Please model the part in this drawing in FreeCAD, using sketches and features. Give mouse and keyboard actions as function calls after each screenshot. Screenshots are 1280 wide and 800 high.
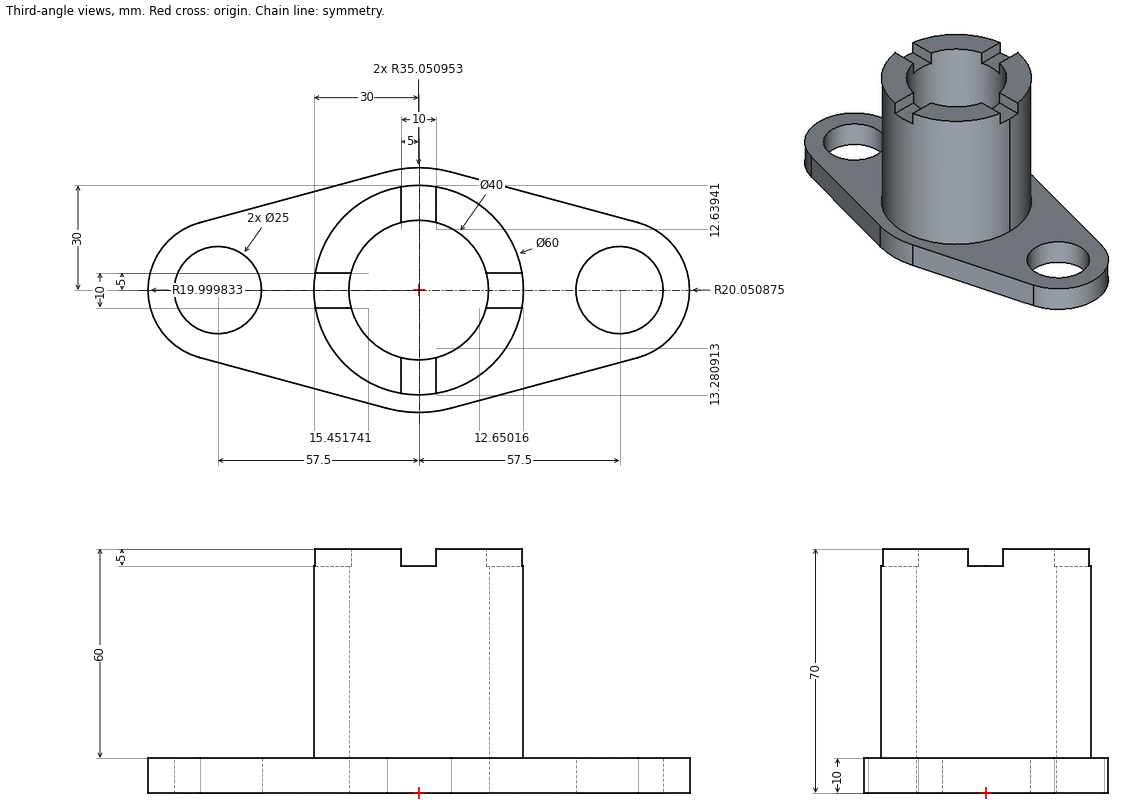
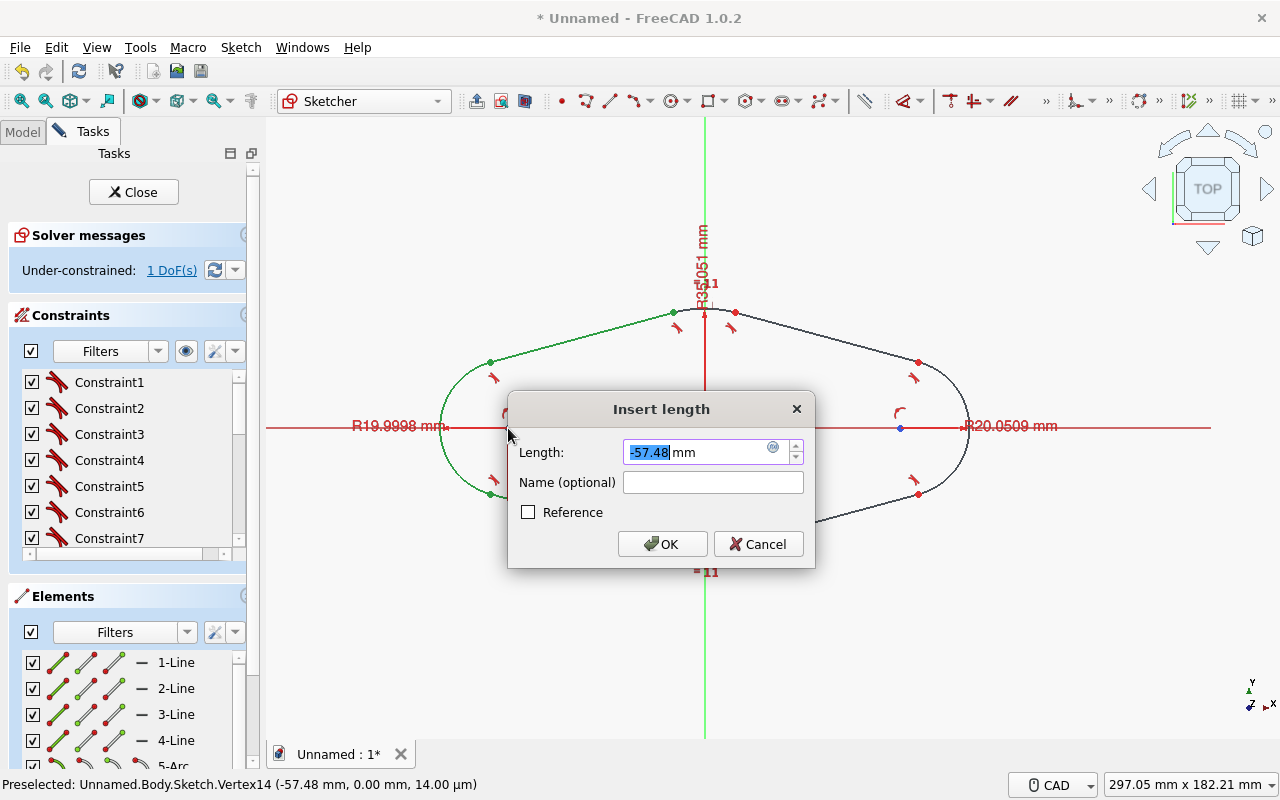
text(-57.5)
key(Return)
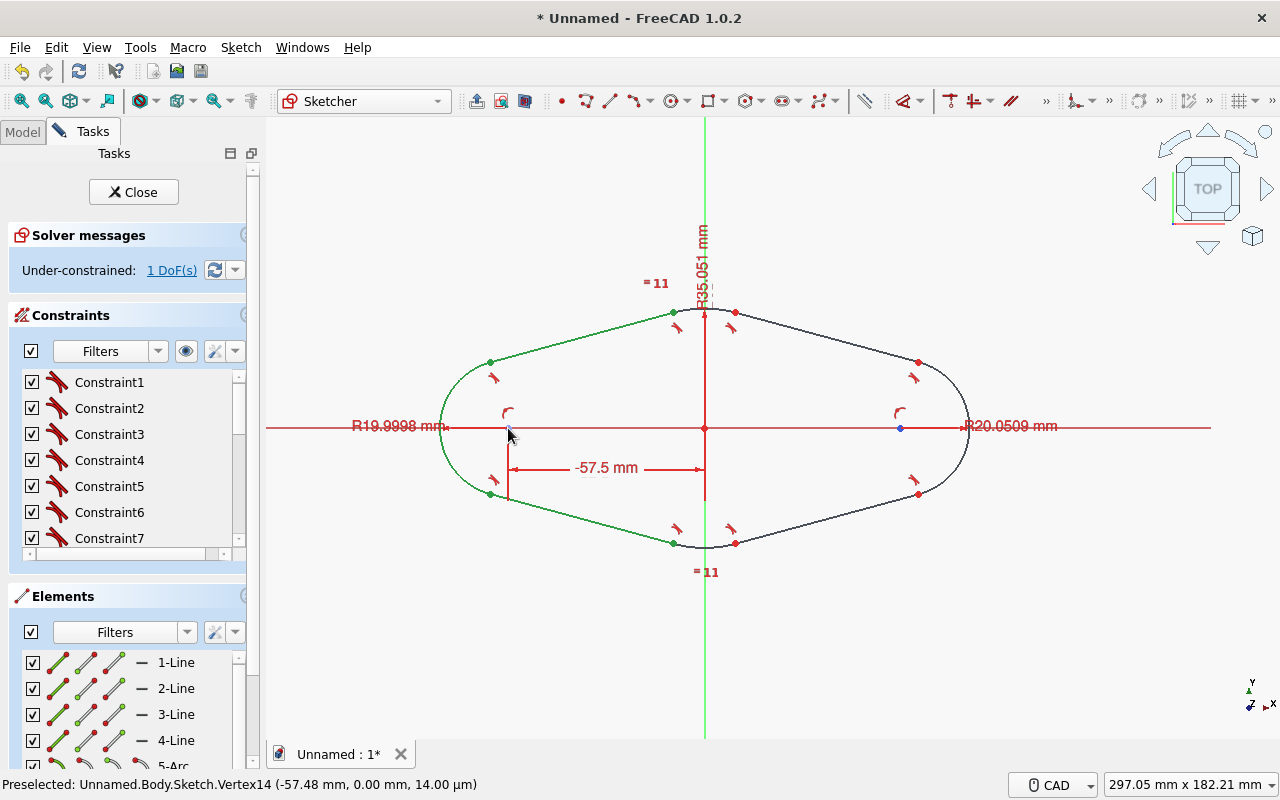
click(901, 428)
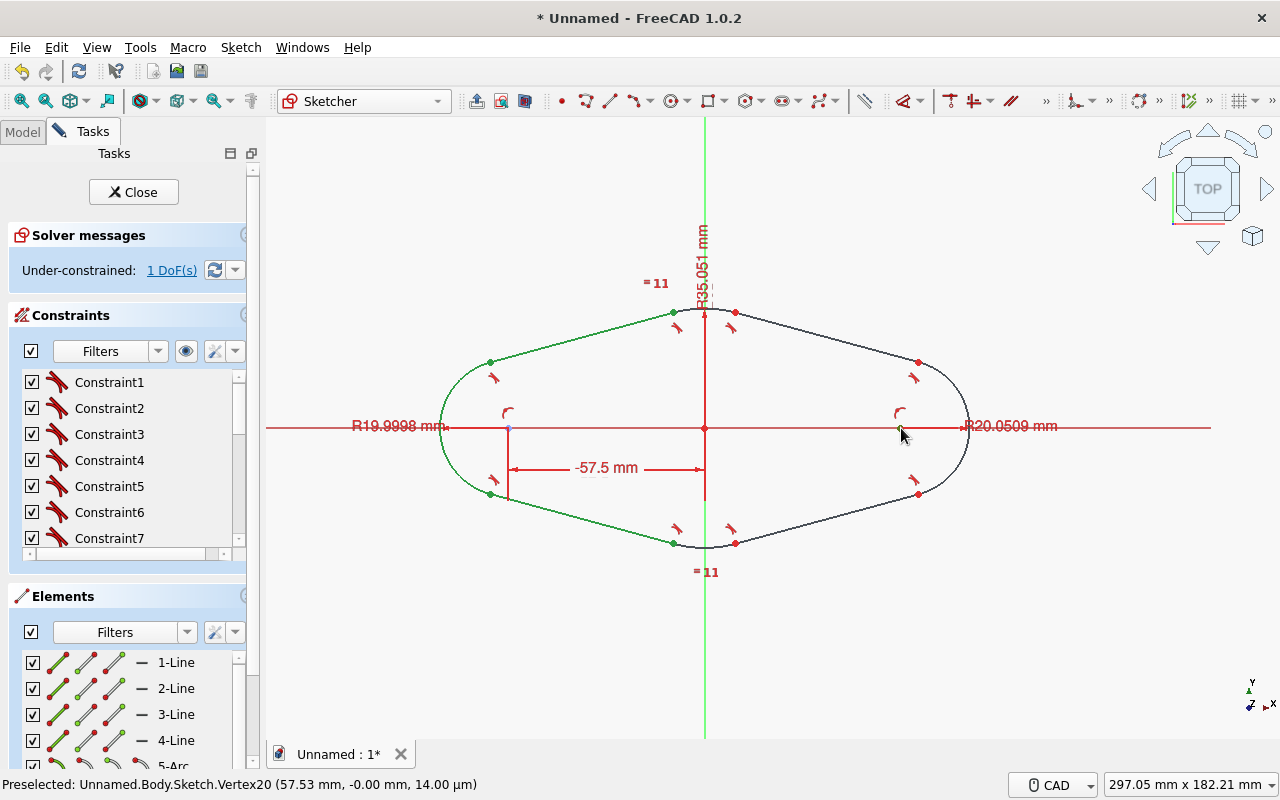
key(l)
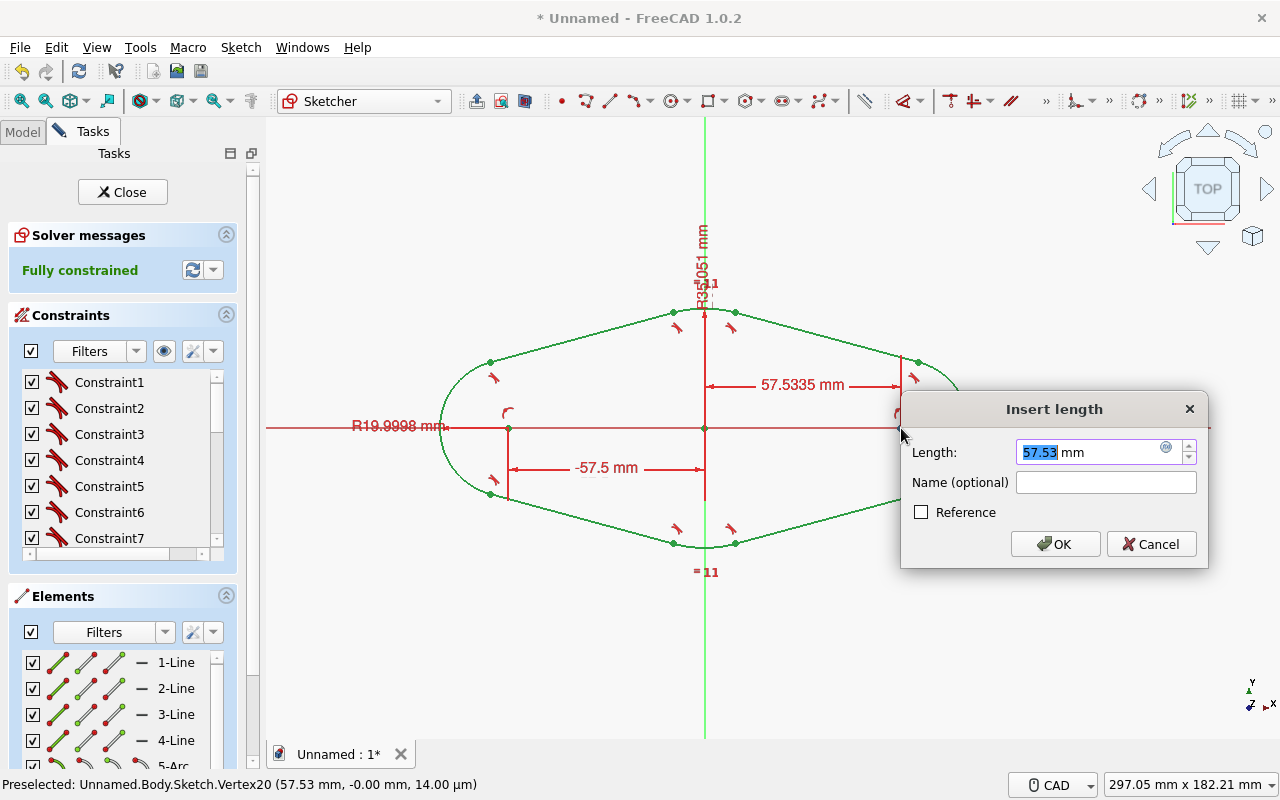
text(57.5)
key(Return)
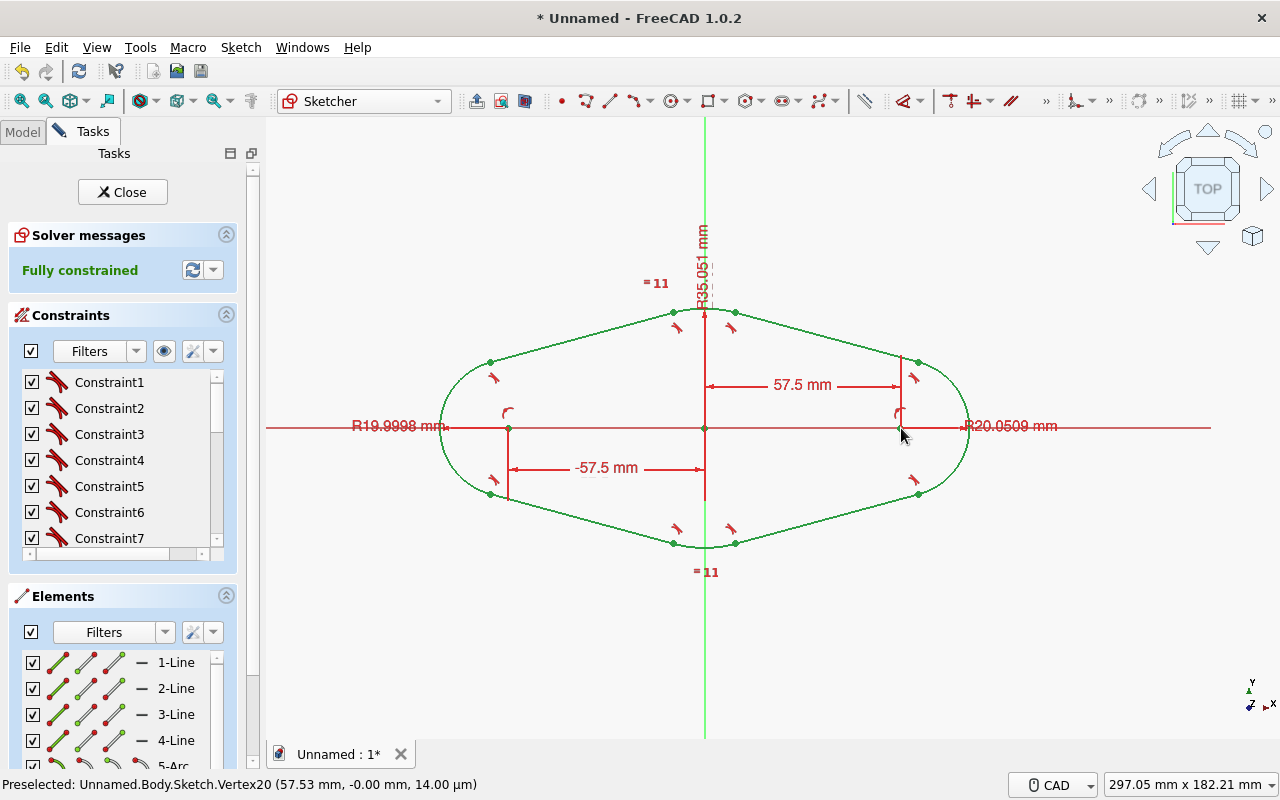
click(123, 192)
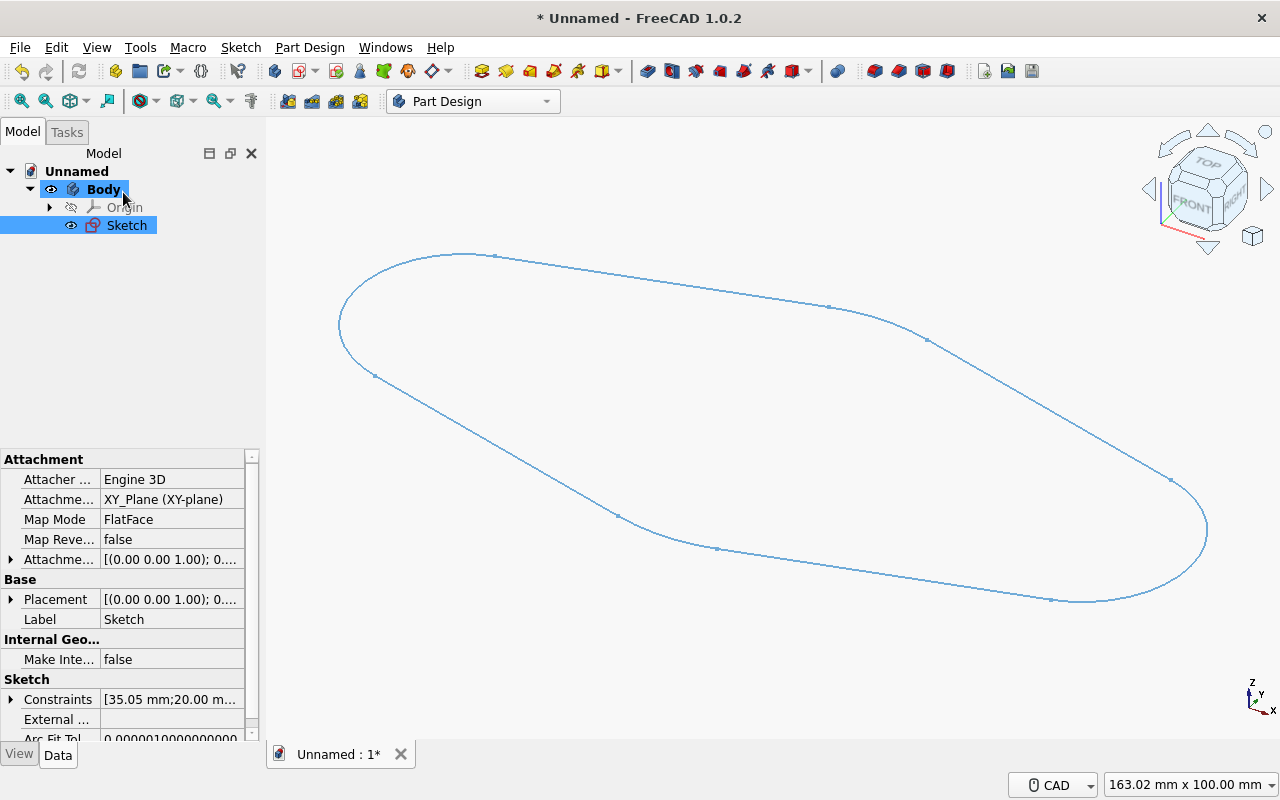
click(482, 72)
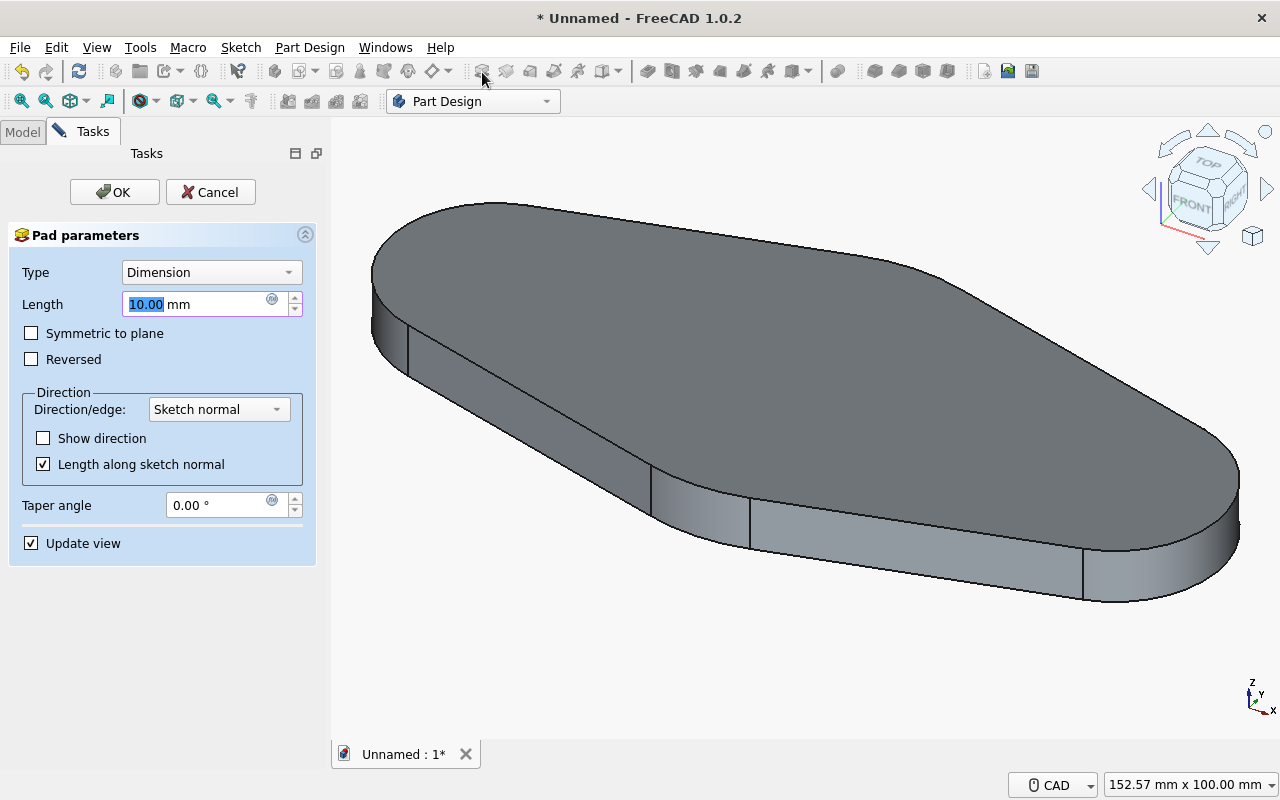
text(10)
key(Tab)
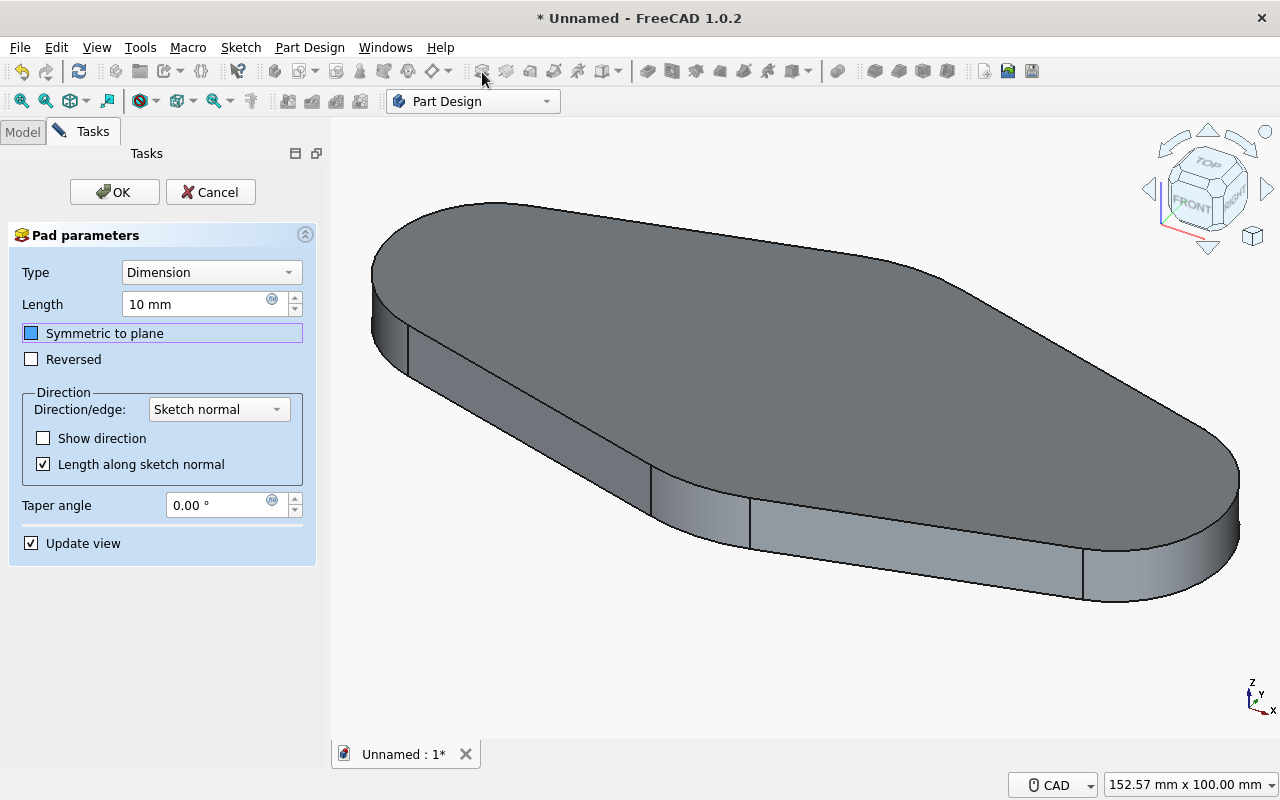
click(115, 192)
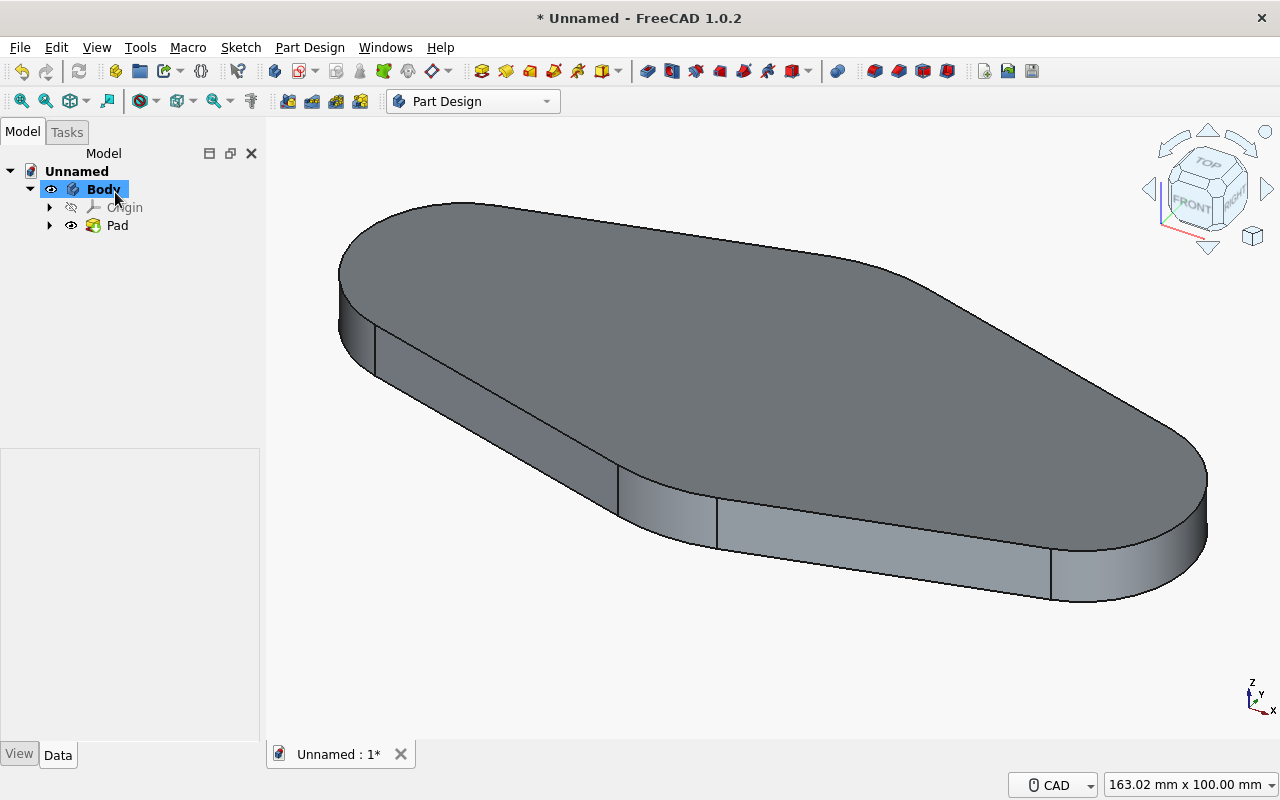
click(22, 102)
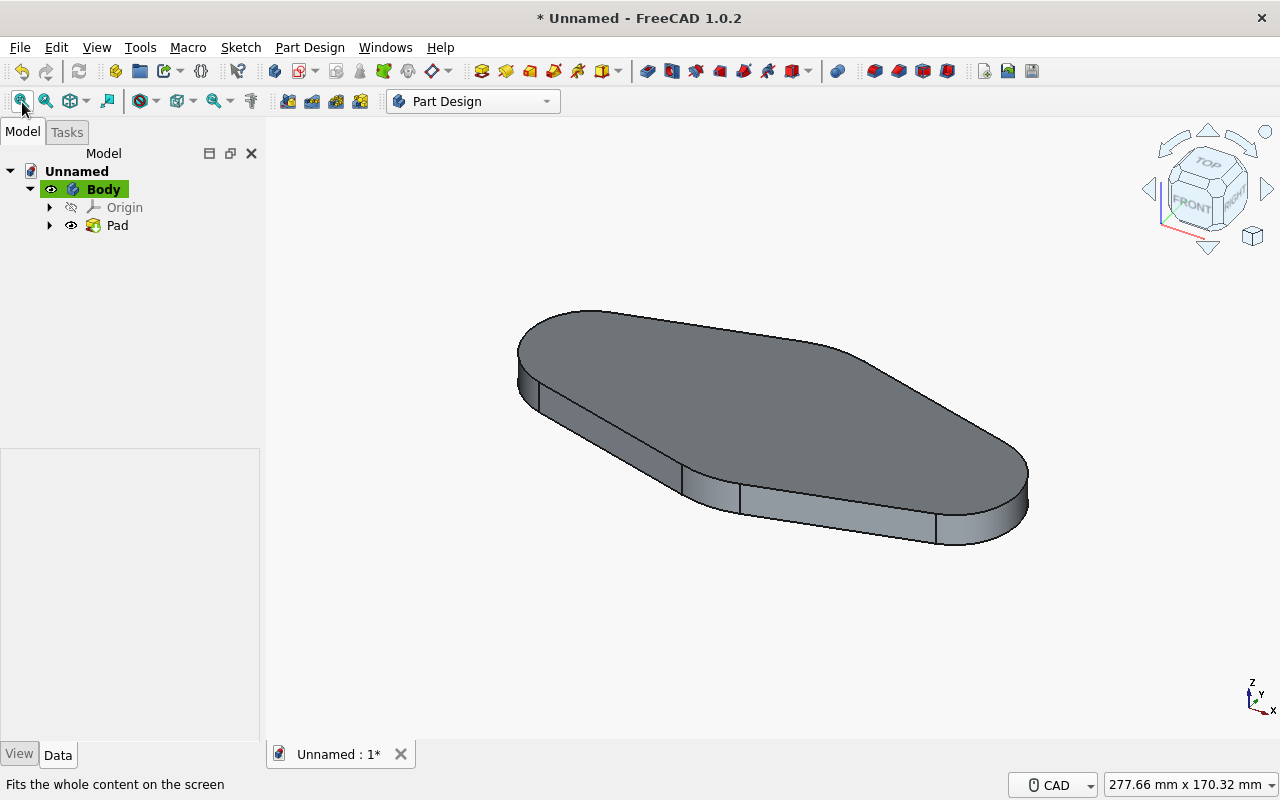
click(773, 412)